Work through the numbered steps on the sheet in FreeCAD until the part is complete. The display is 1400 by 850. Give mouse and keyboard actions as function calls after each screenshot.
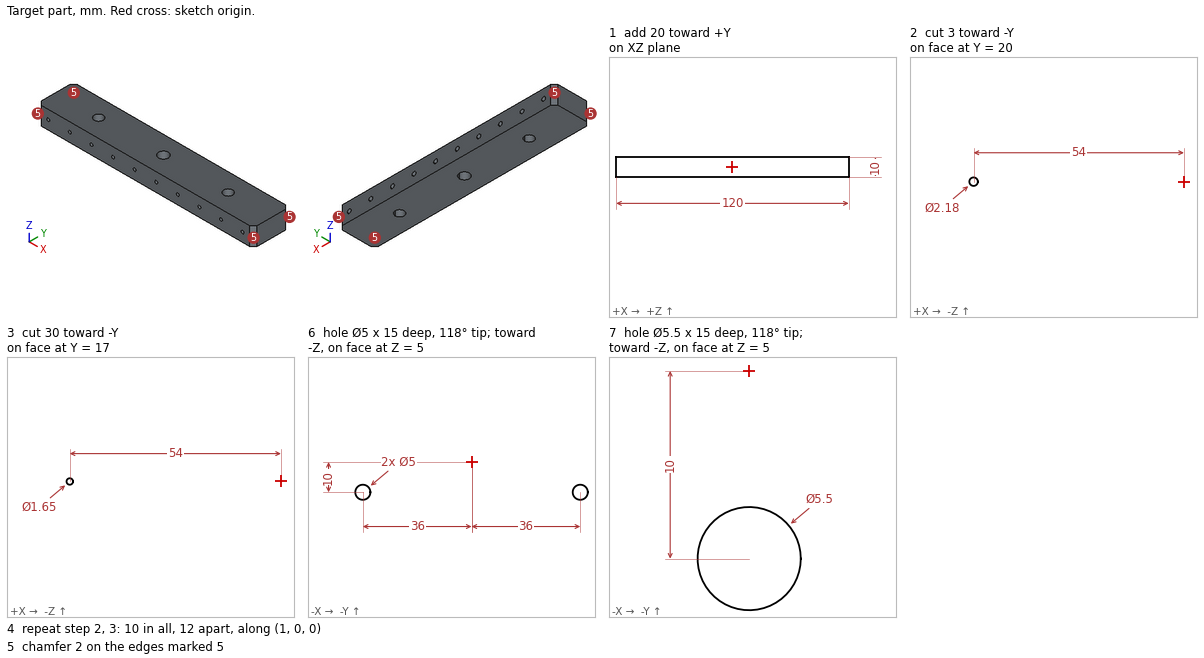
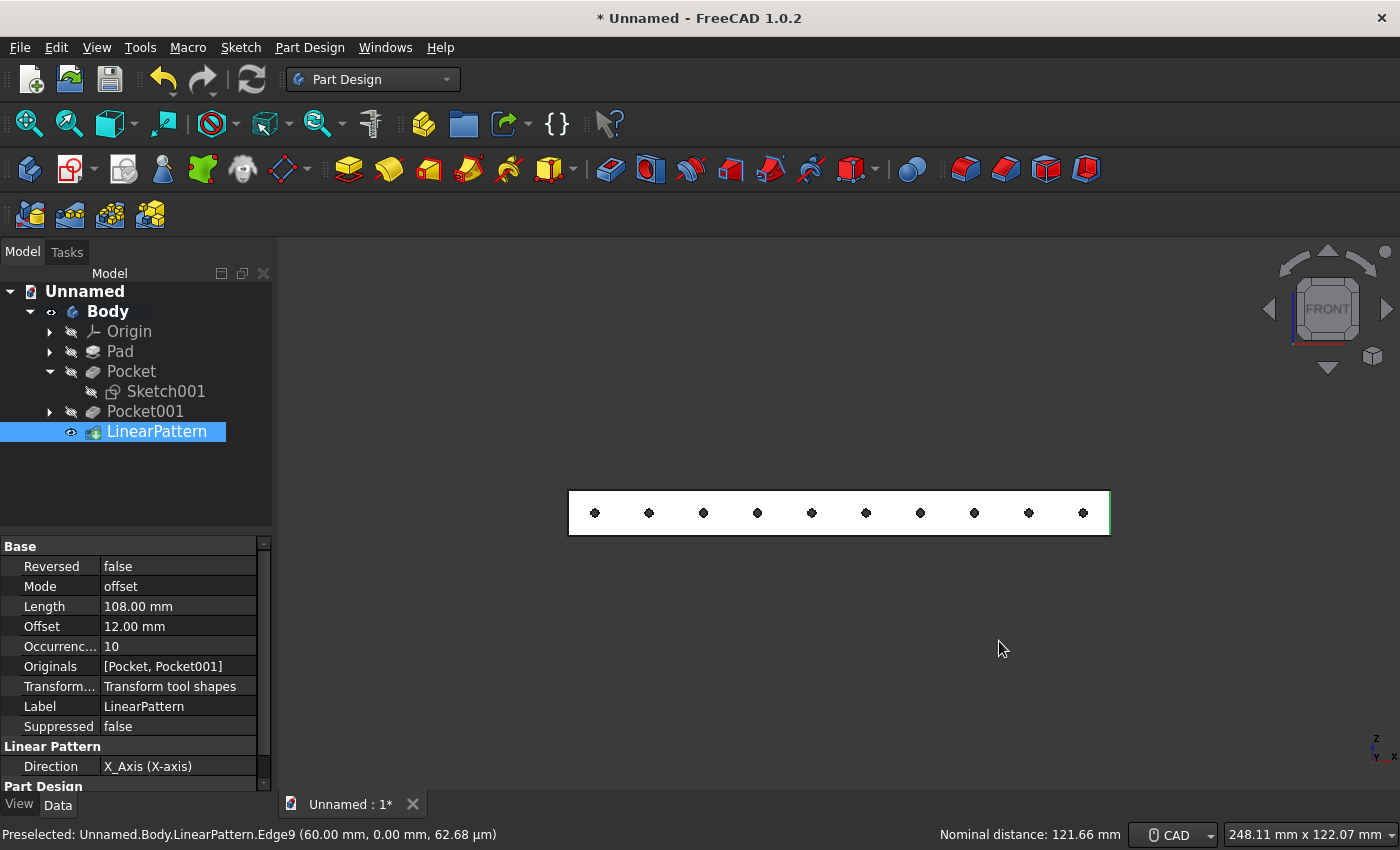
click(568, 512, ctrl)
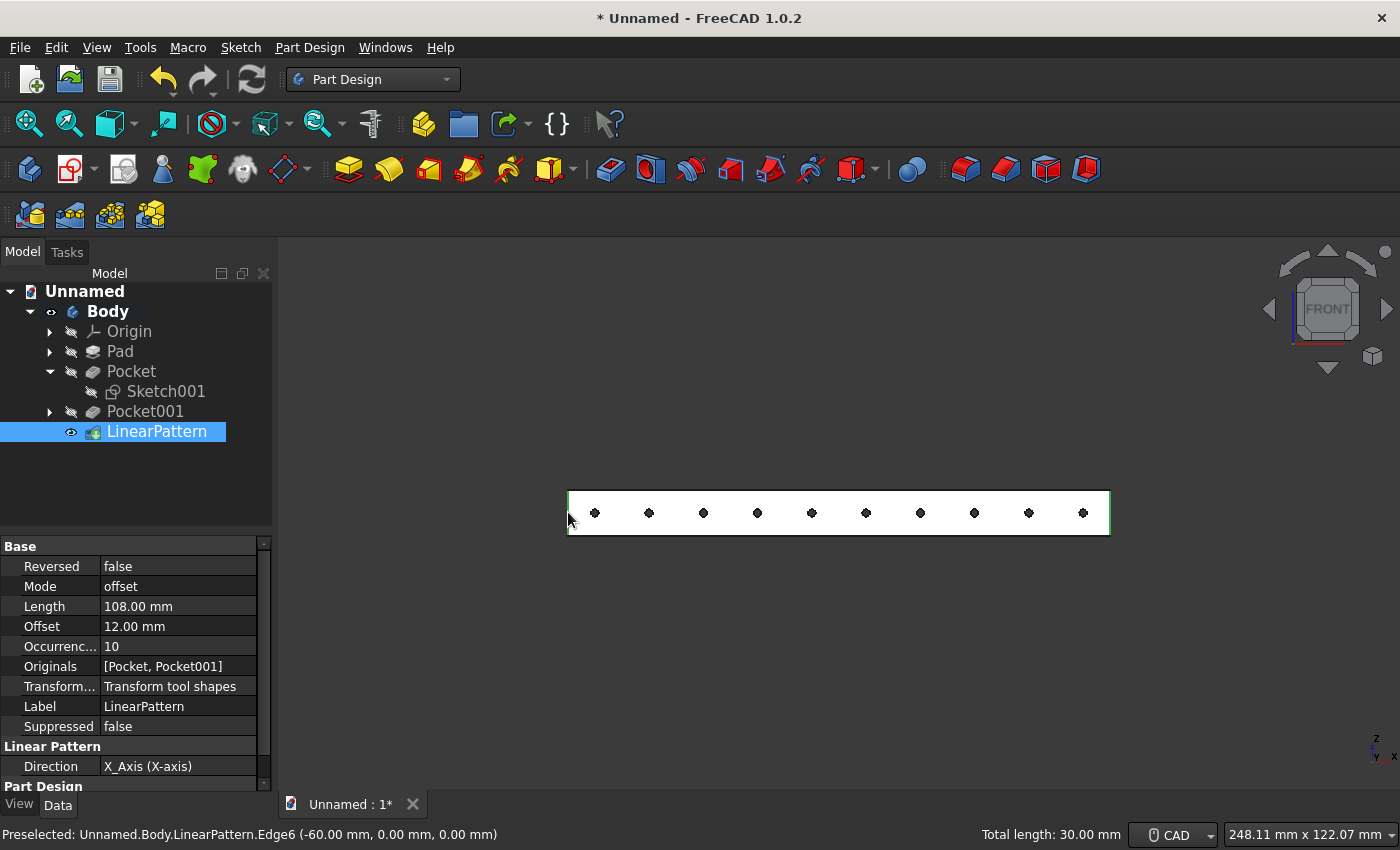
key(3)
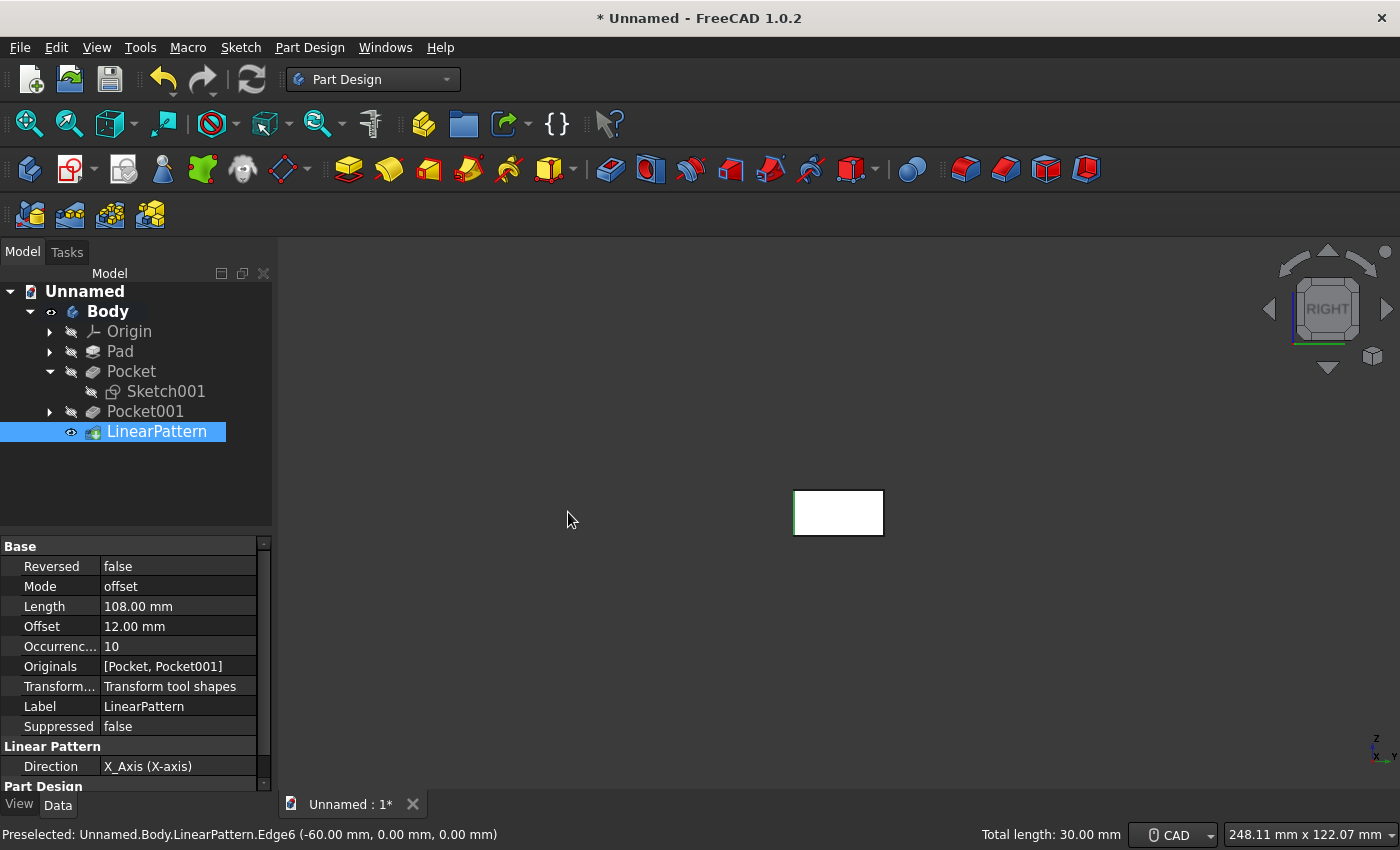
click(30, 124)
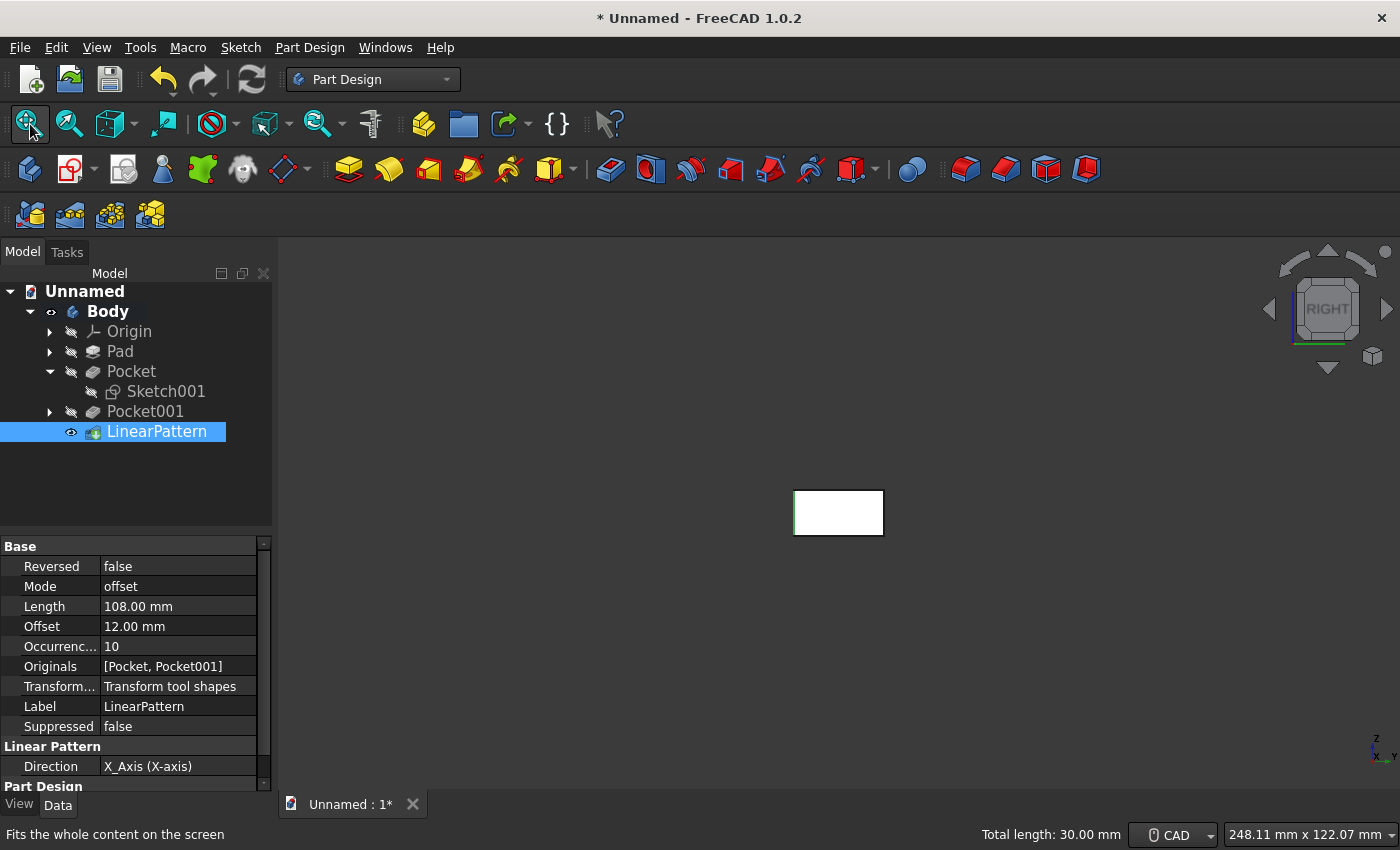
click(884, 512, ctrl)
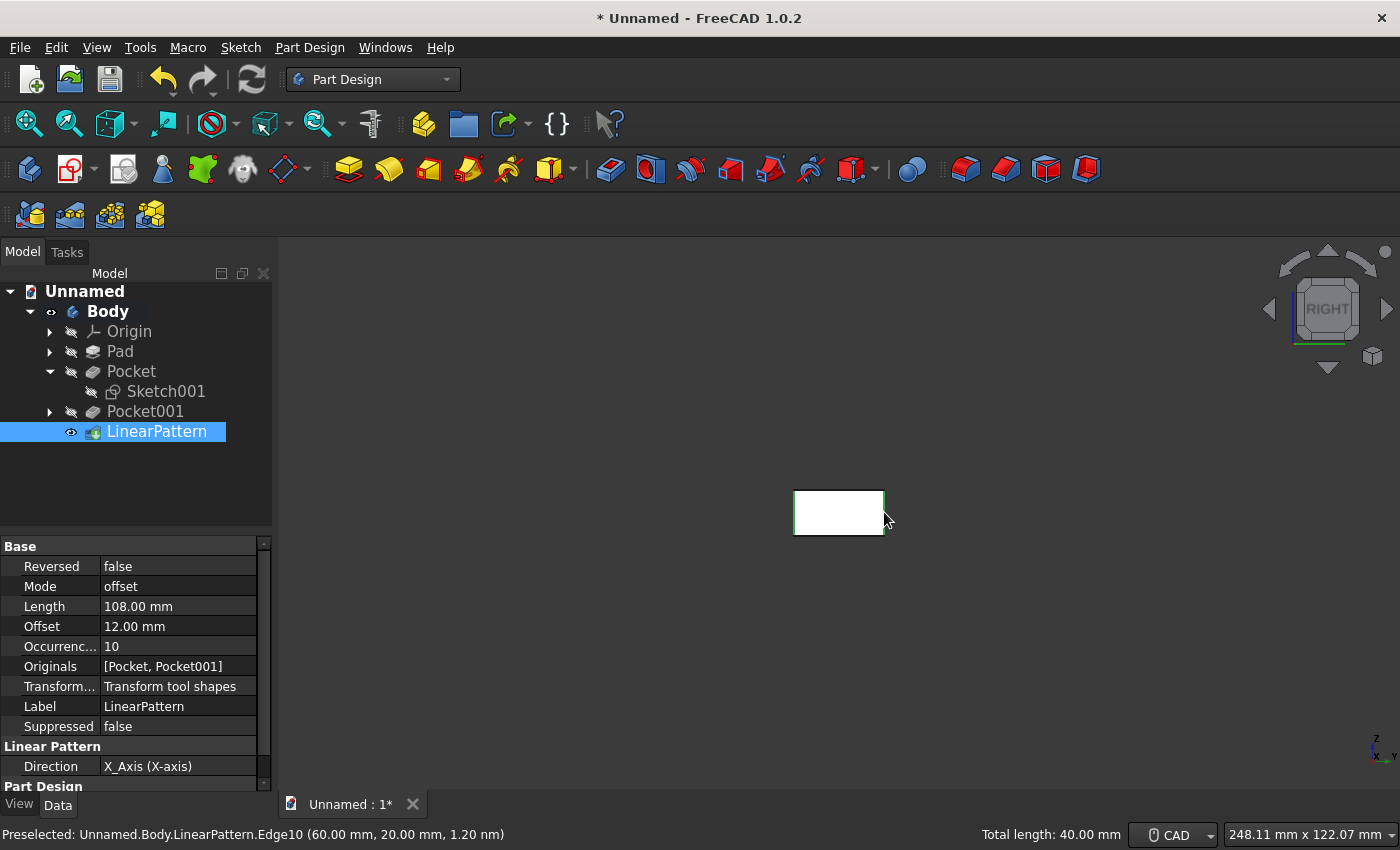
click(1006, 170)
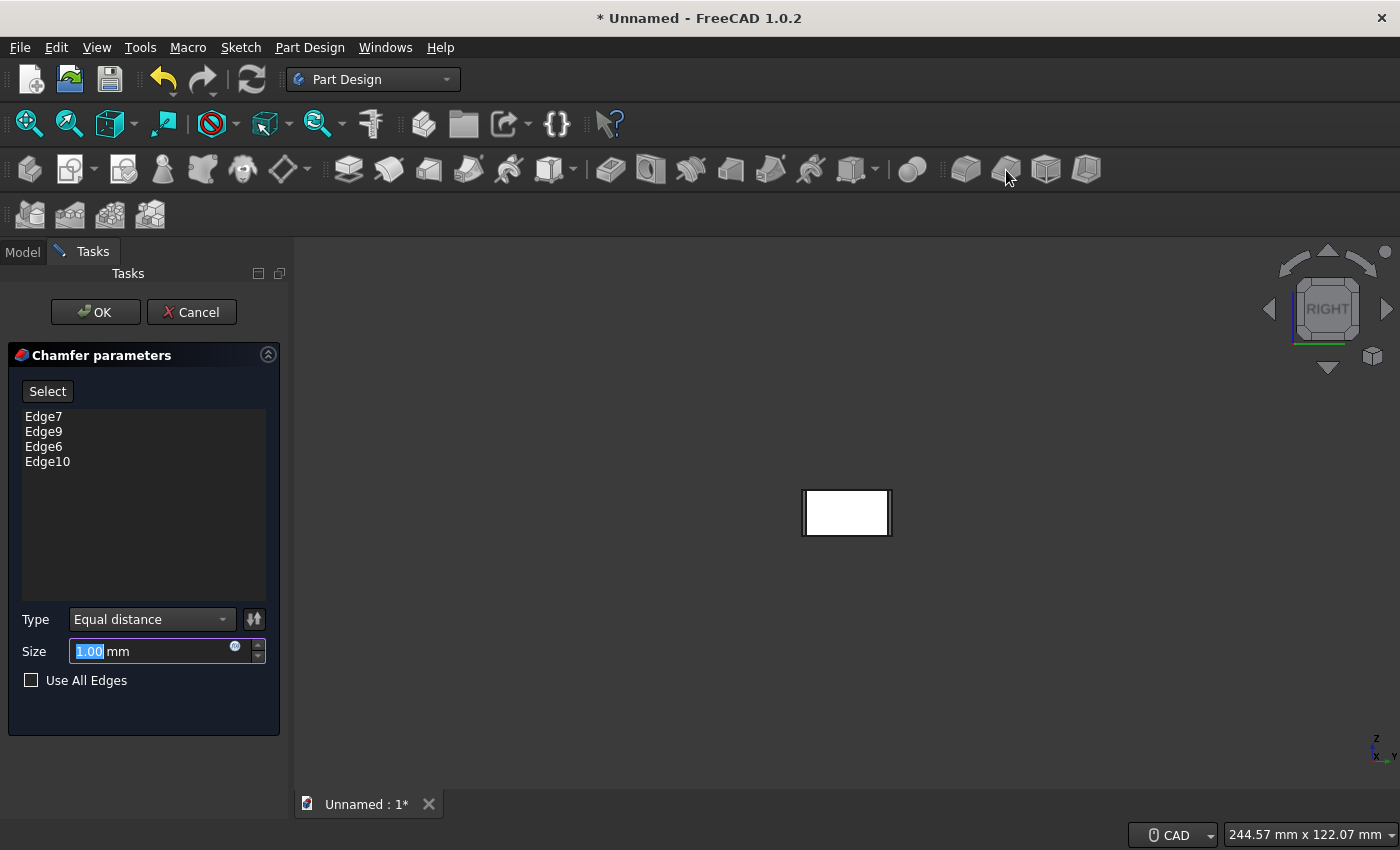
text(2)
key(Tab)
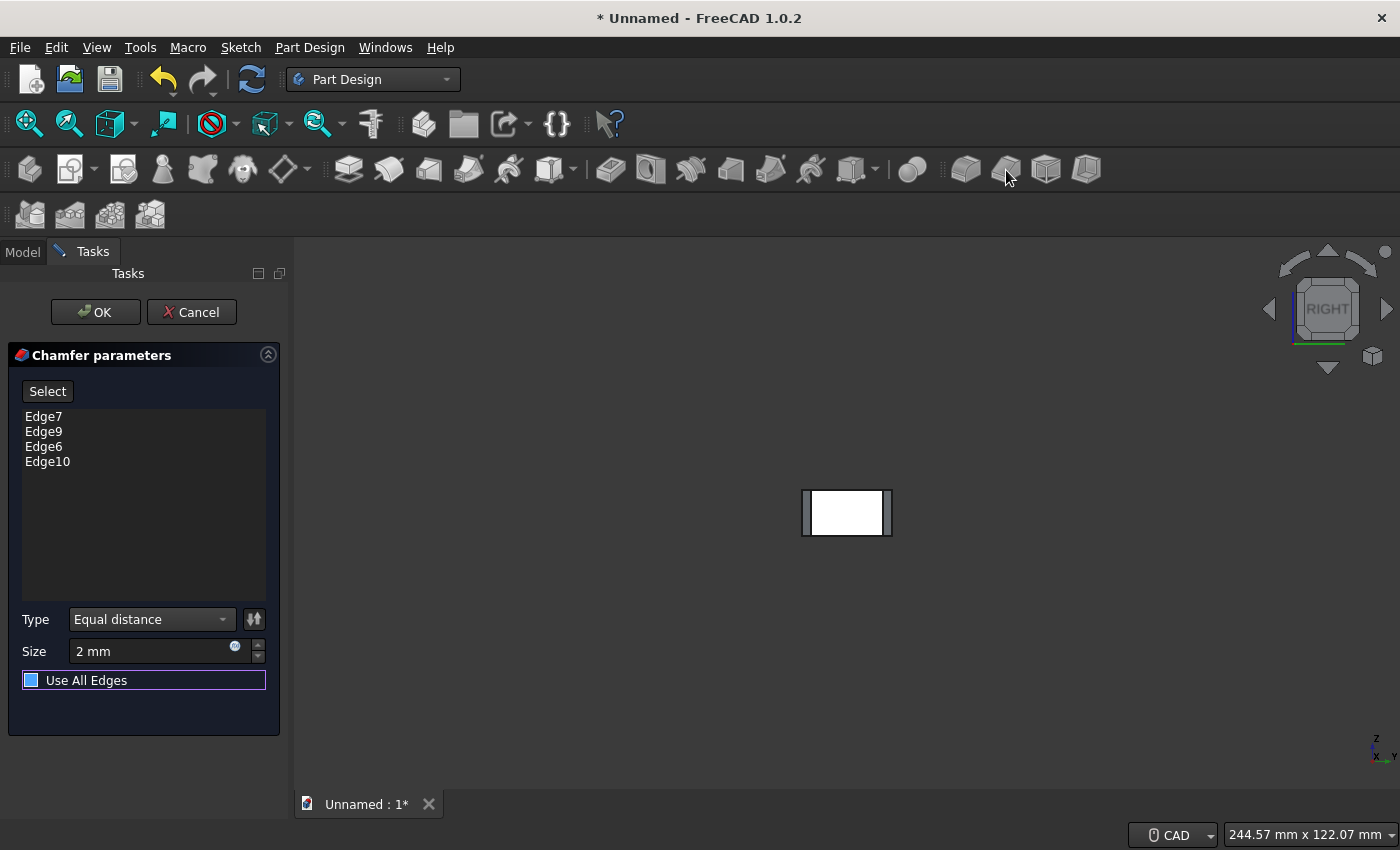
click(96, 312)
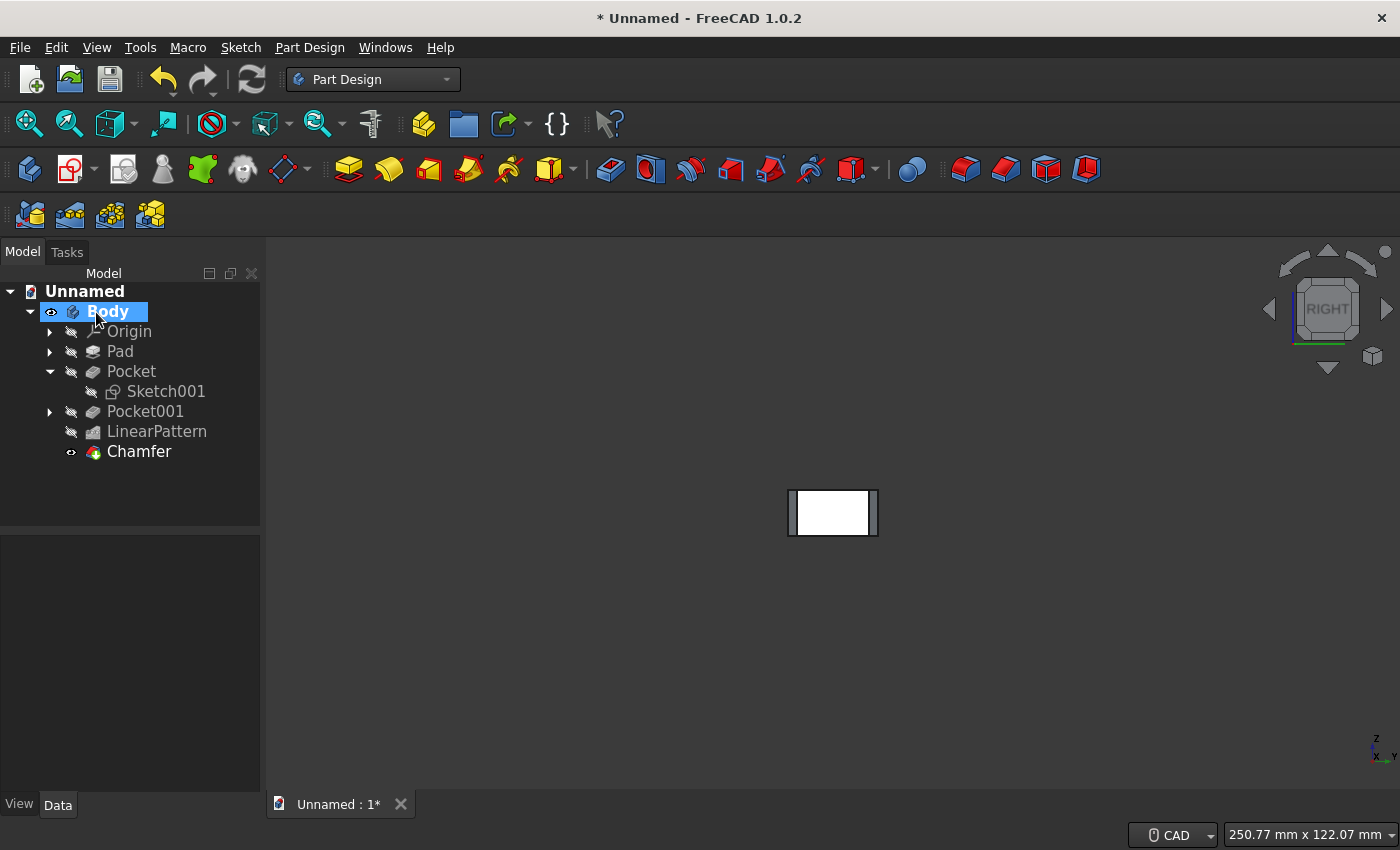
click(30, 124)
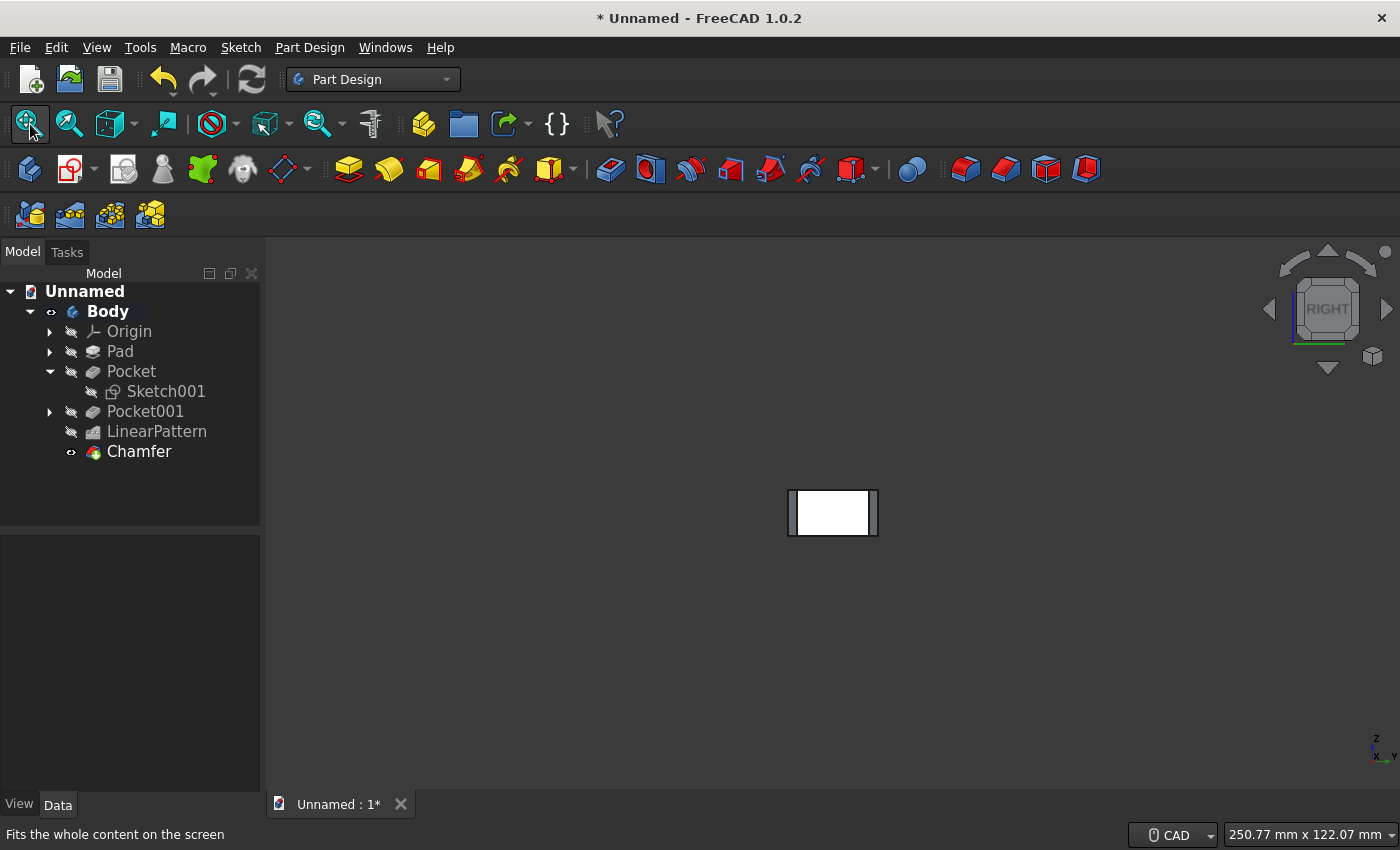
key(0)